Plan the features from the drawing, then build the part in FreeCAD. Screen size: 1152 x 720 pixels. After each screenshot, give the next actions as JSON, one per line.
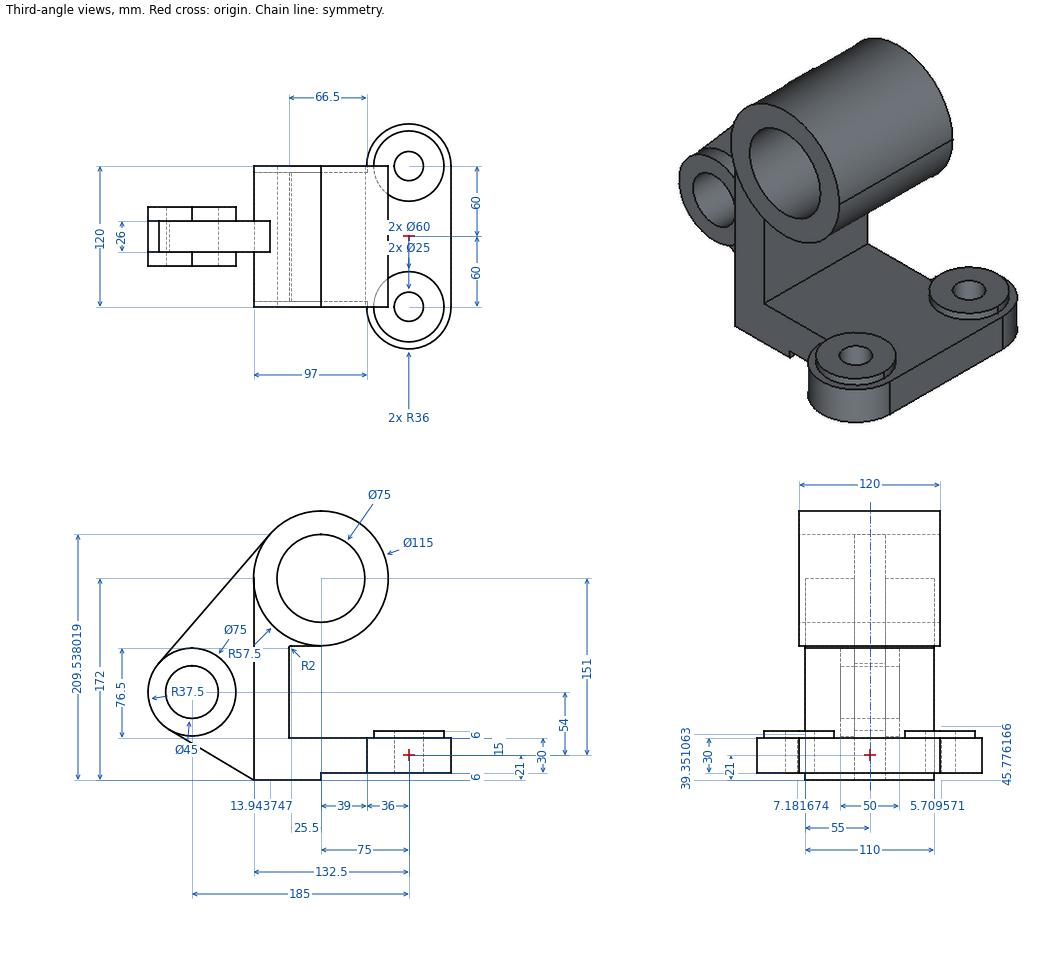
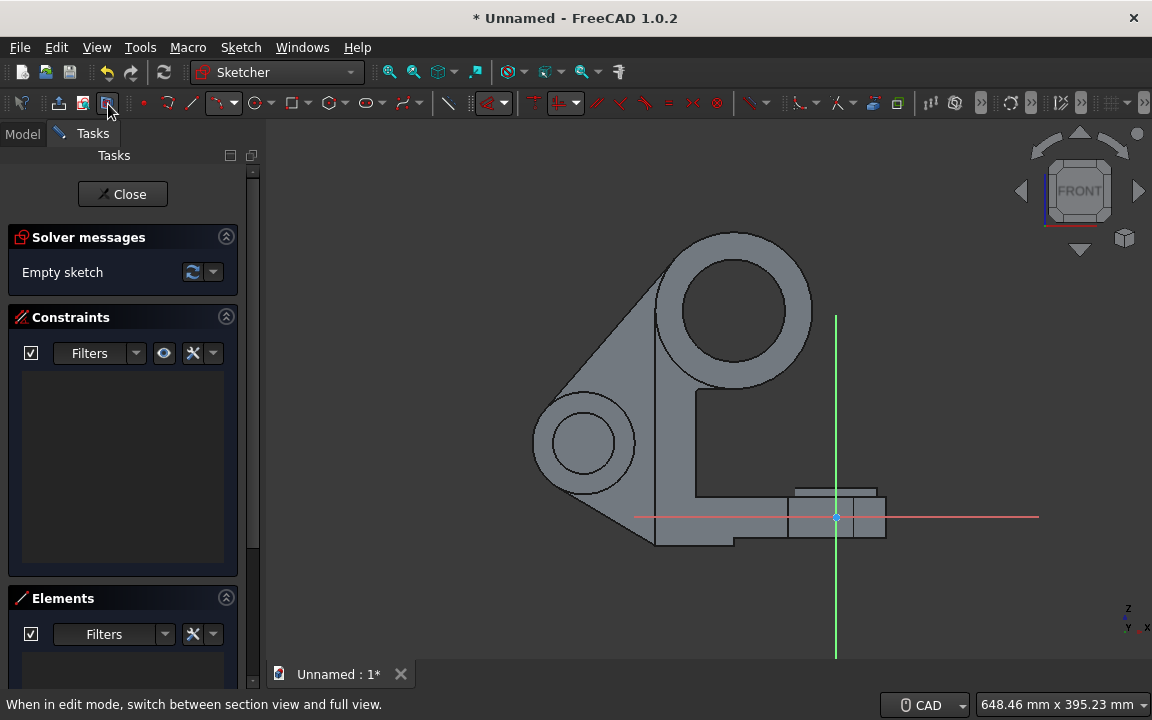
{"action": "scroll", "coordinate": [572, 454], "scroll_direction": "up", "scroll_amount": 9}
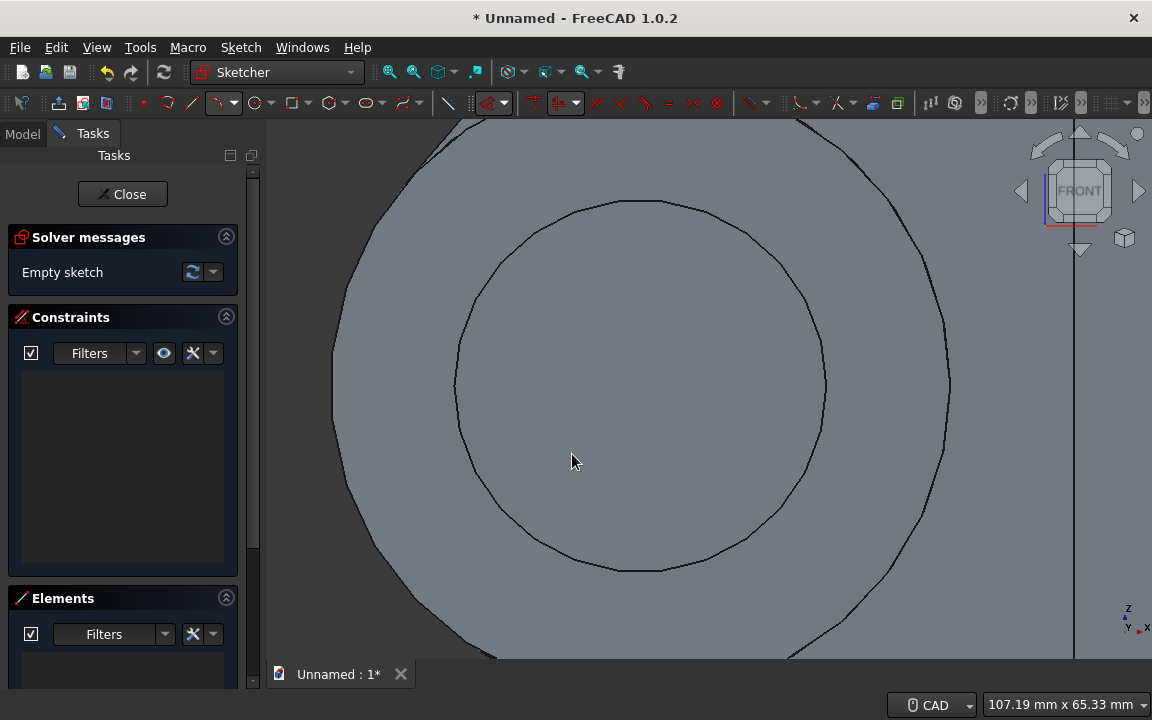
{"action": "left_click", "coordinate": [256, 104]}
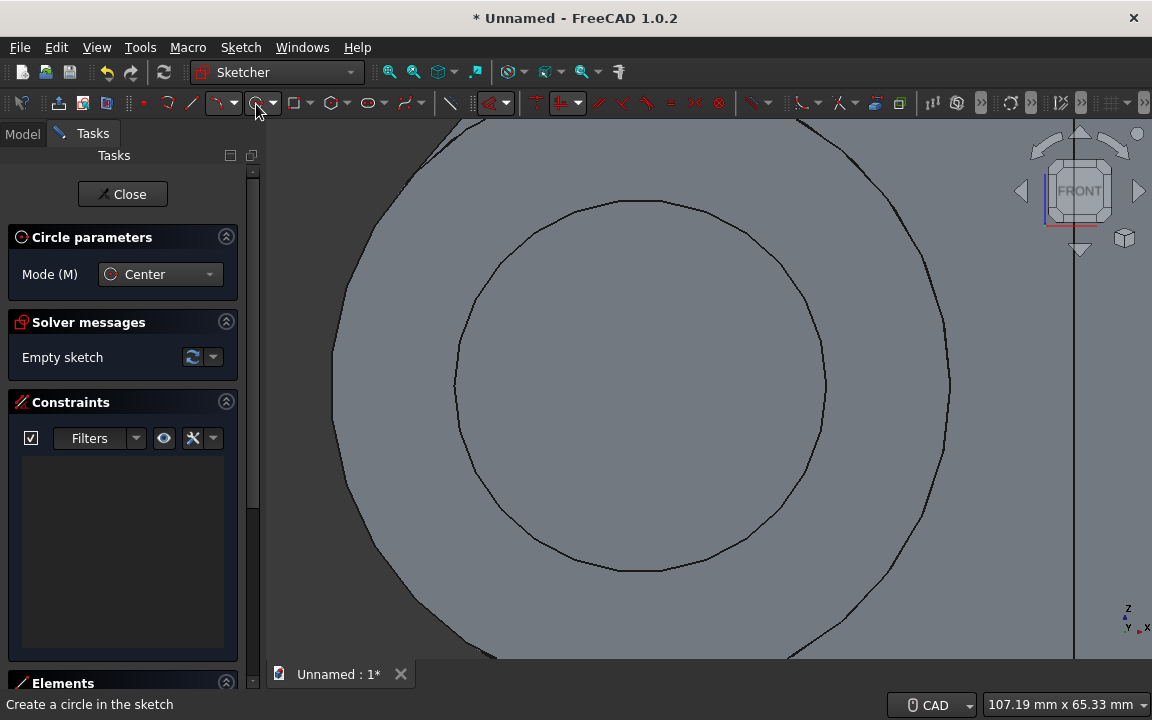
{"action": "left_click", "coordinate": [640, 386]}
{"action": "left_click", "coordinate": [772, 254]}
{"action": "key", "text": "Escape"}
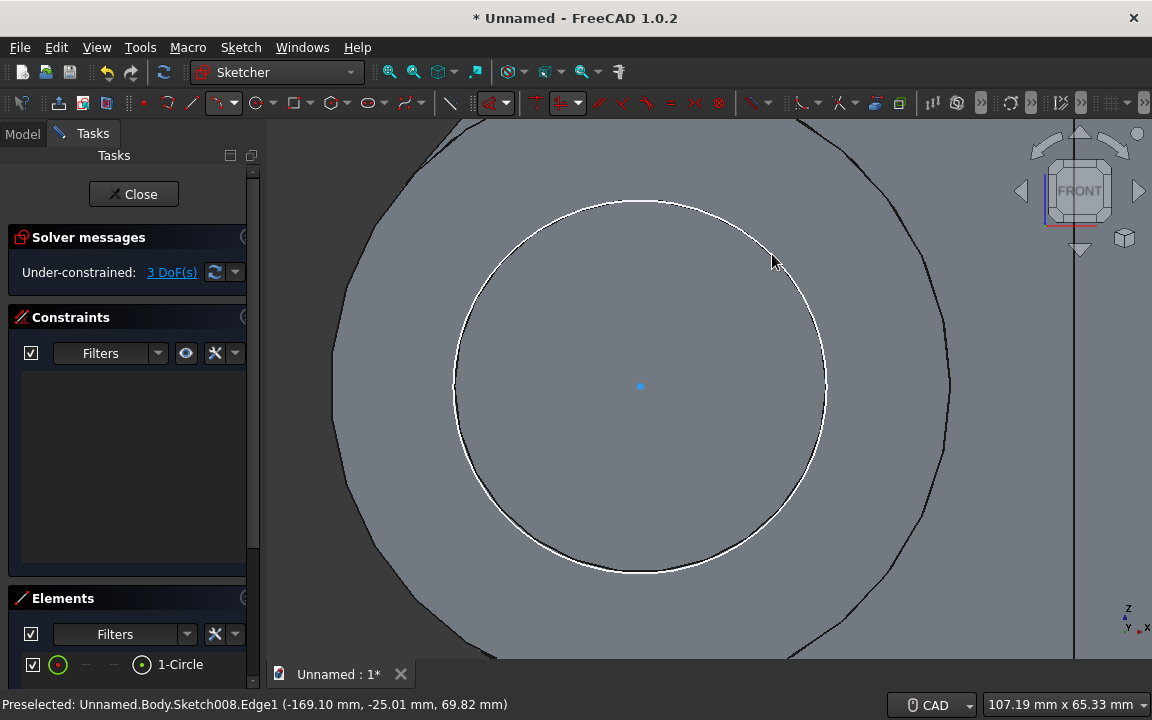
{"action": "left_click", "coordinate": [772, 255]}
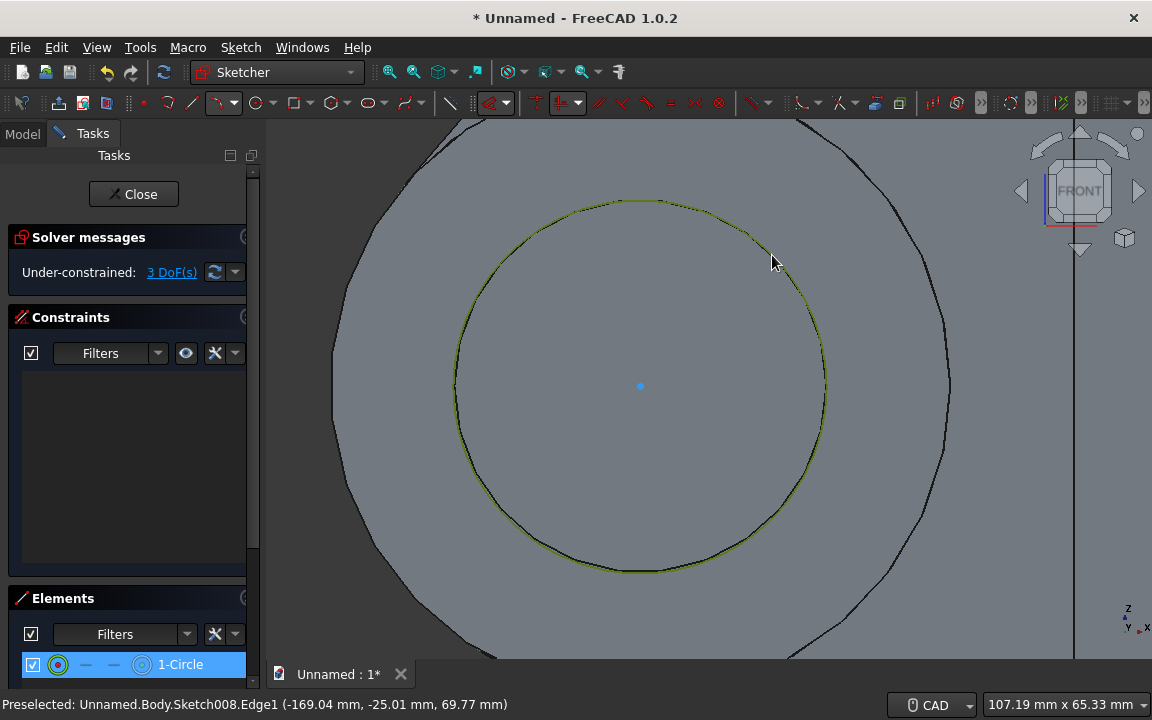
{"action": "key", "text": "k o"}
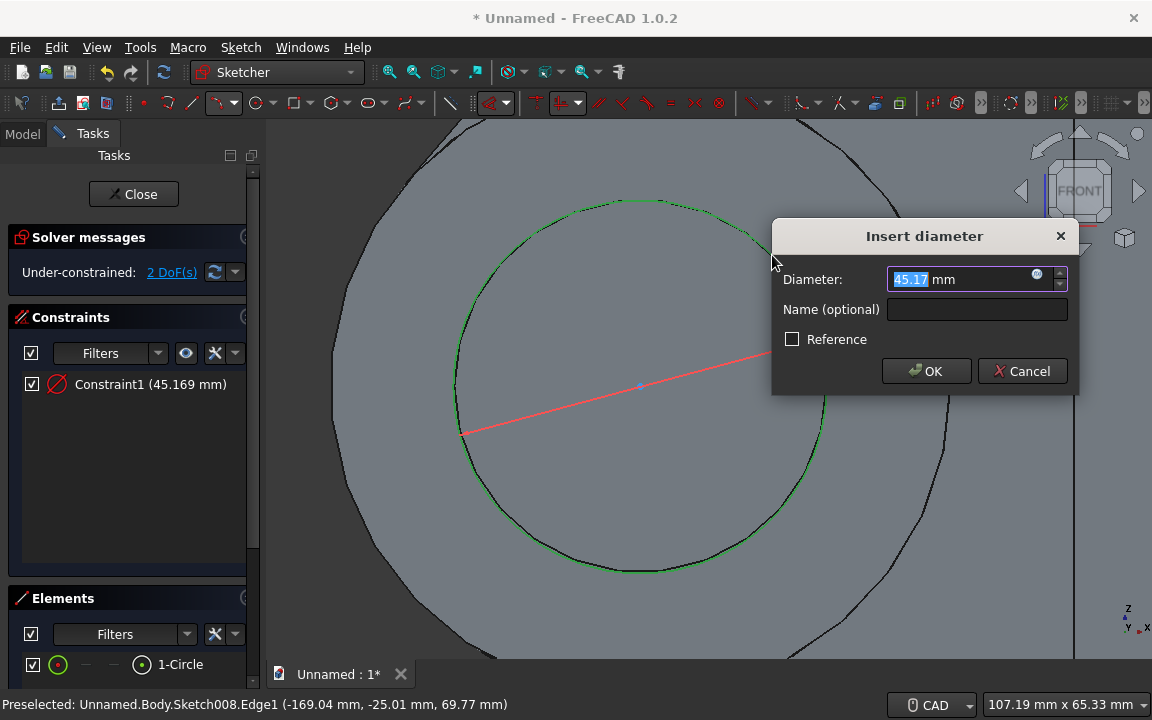
{"action": "type", "text": "45"}
{"action": "key", "text": "Return"}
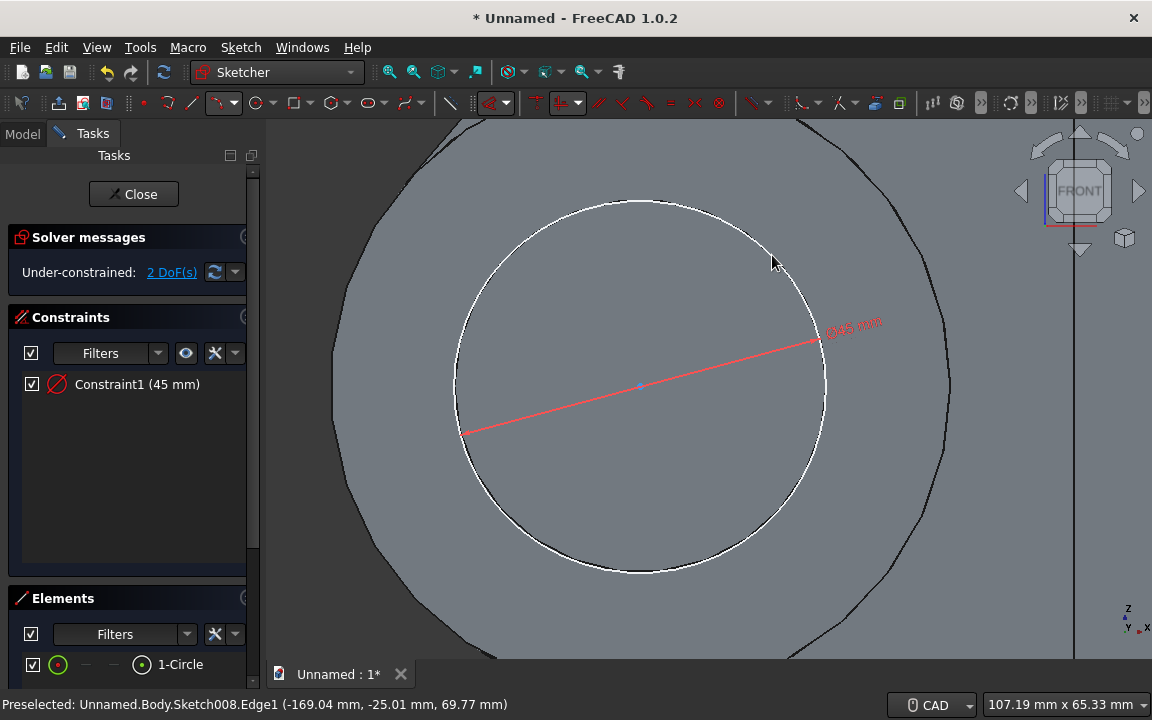
{"action": "left_click", "coordinate": [640, 387]}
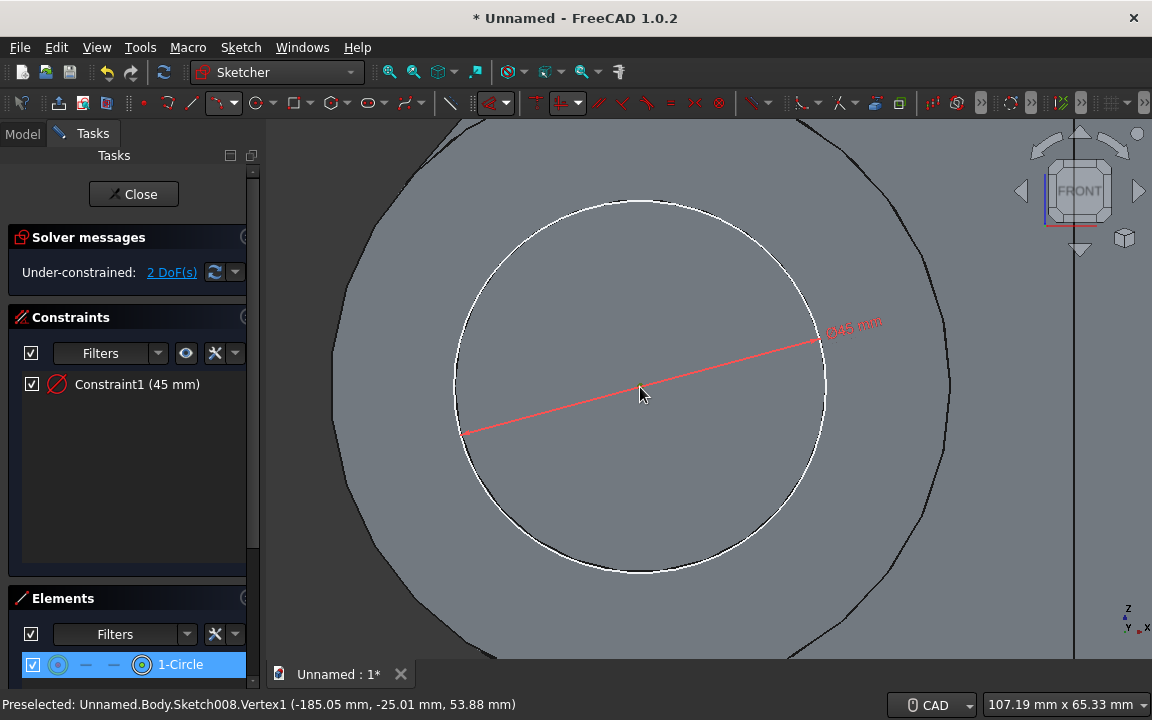
{"action": "key", "text": "i"}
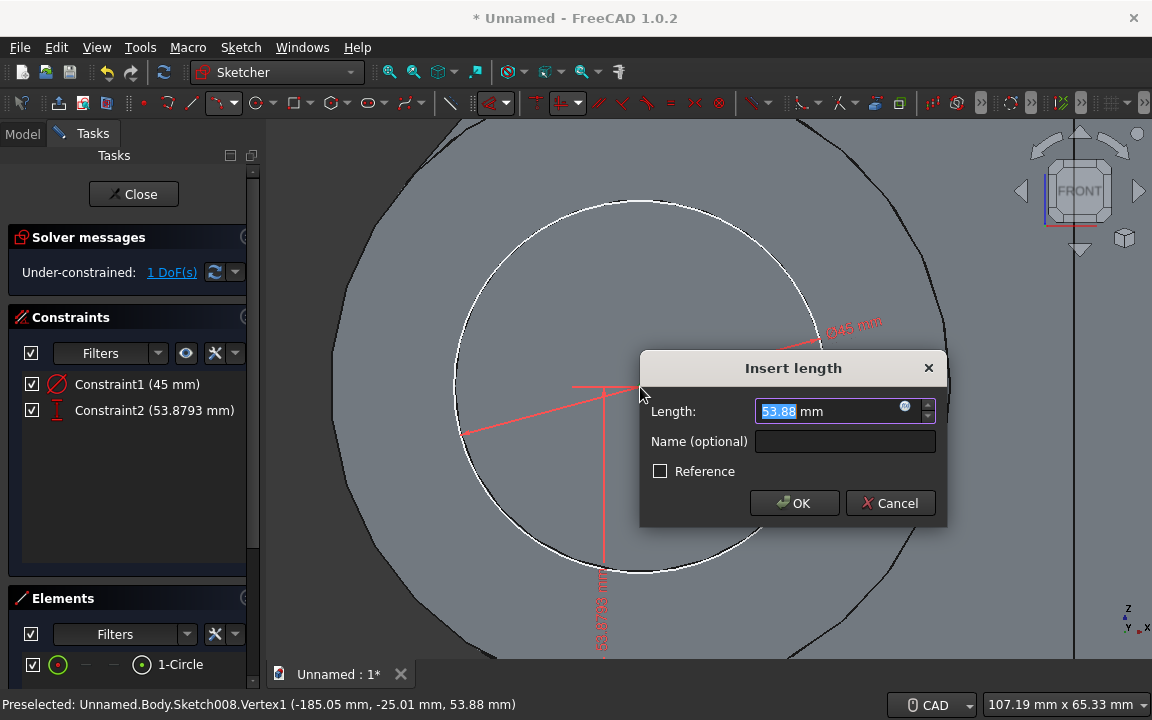
{"action": "type", "text": "54"}
{"action": "key", "text": "Return"}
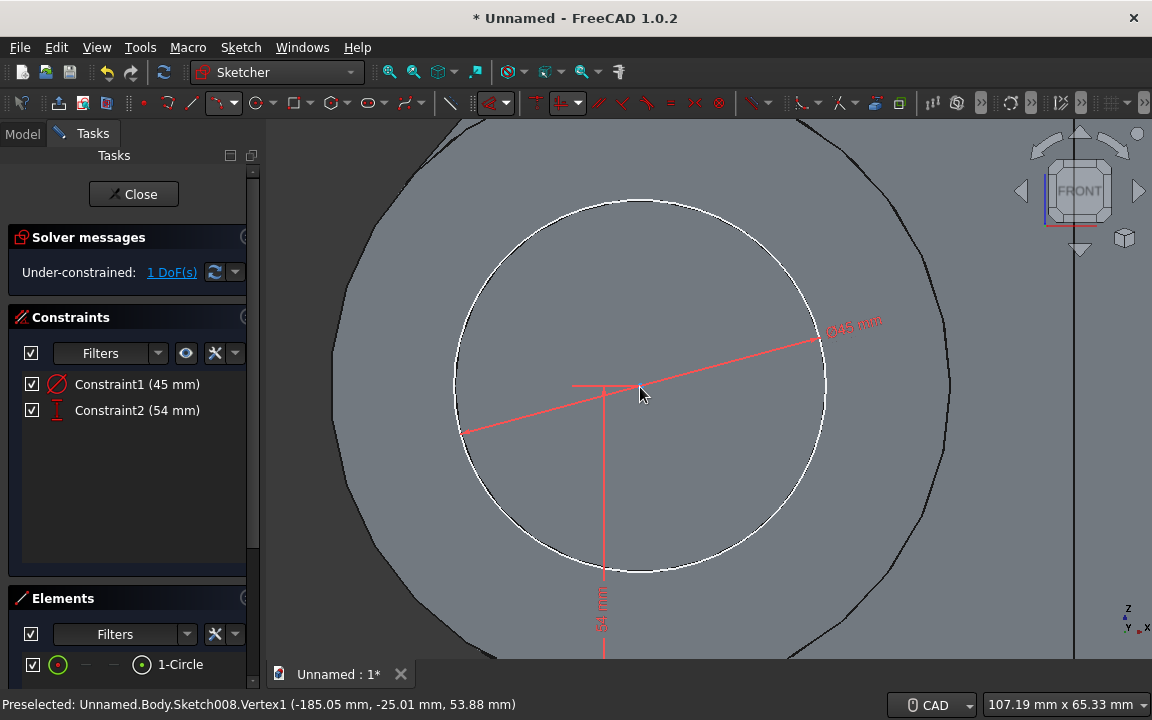
{"action": "left_click", "coordinate": [640, 386]}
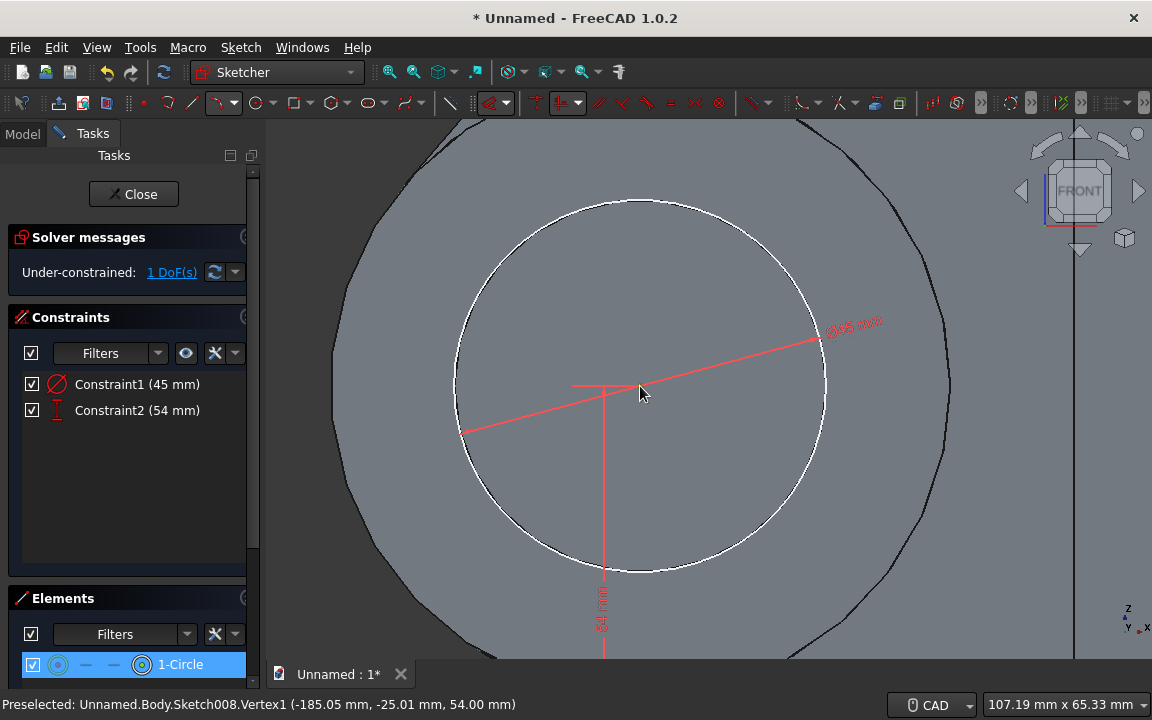
{"action": "left_click", "coordinate": [508, 104]}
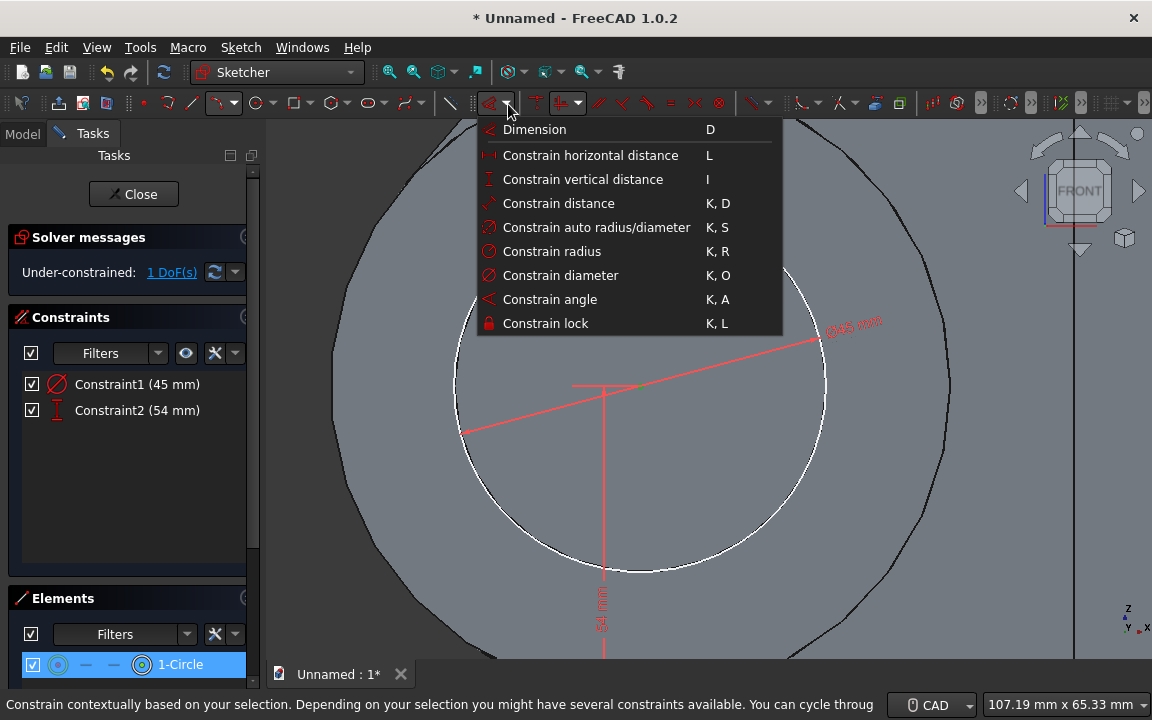
{"action": "left_click", "coordinate": [630, 155]}